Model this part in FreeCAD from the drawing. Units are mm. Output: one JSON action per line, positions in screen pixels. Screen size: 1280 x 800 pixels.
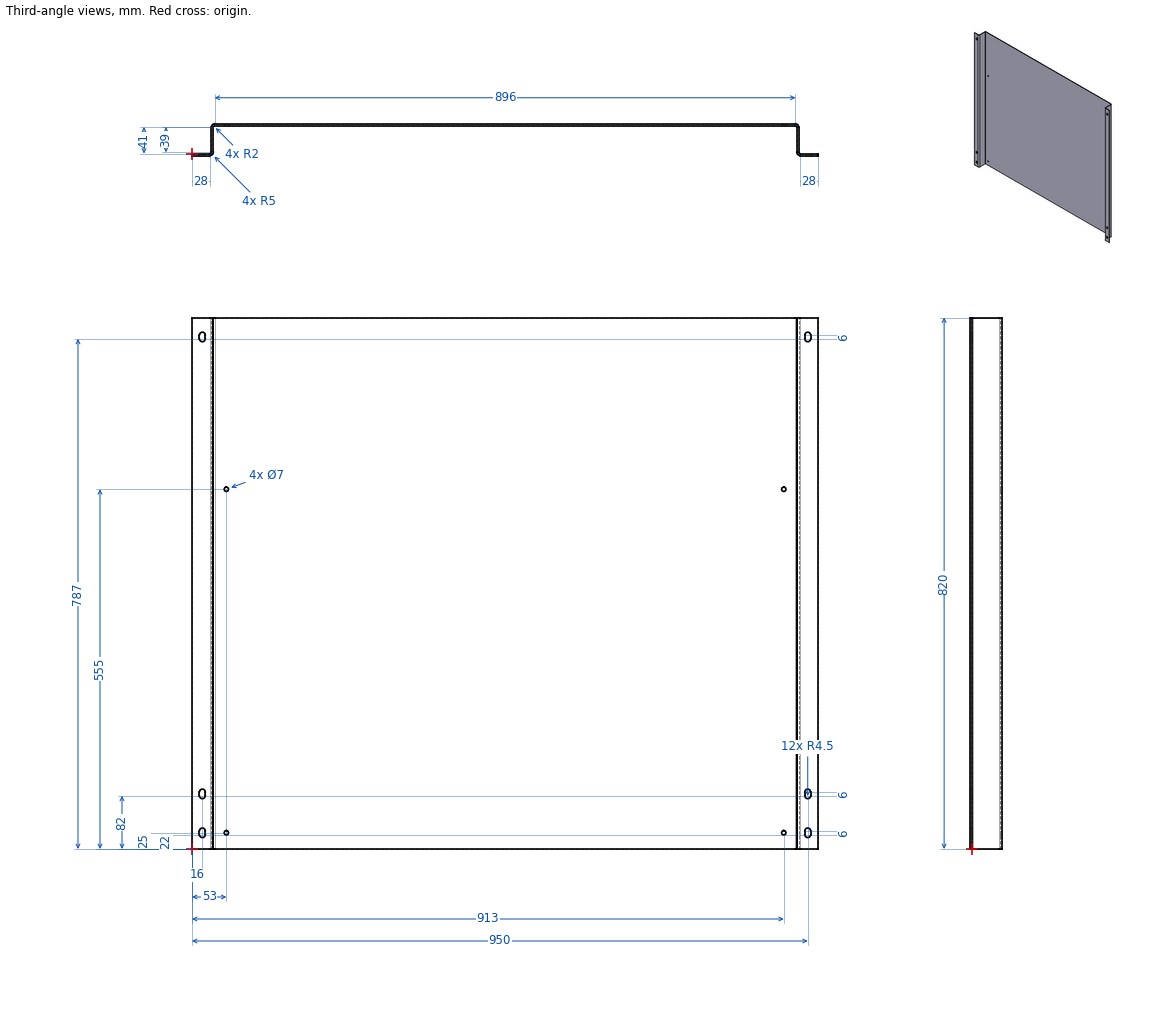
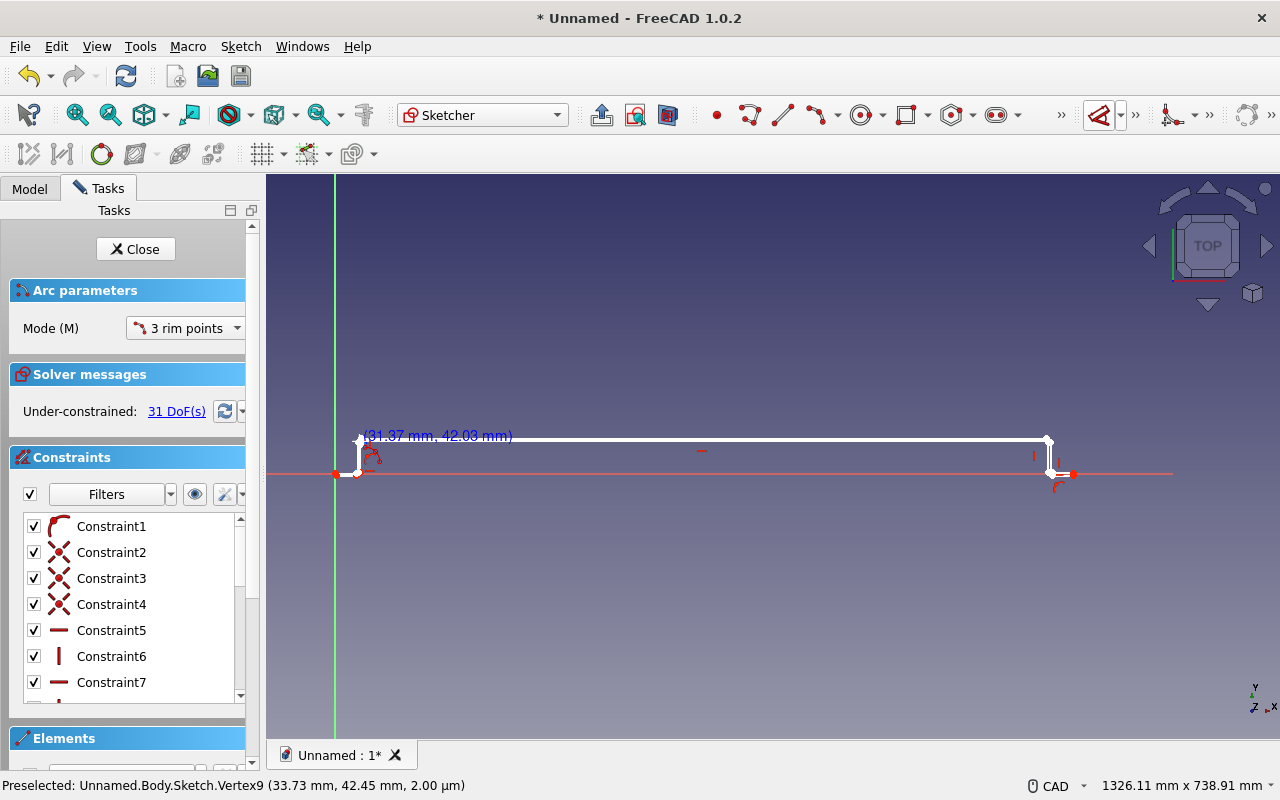
{"action": "scroll", "coordinate": [1047, 441], "scroll_direction": "up", "scroll_amount": 10}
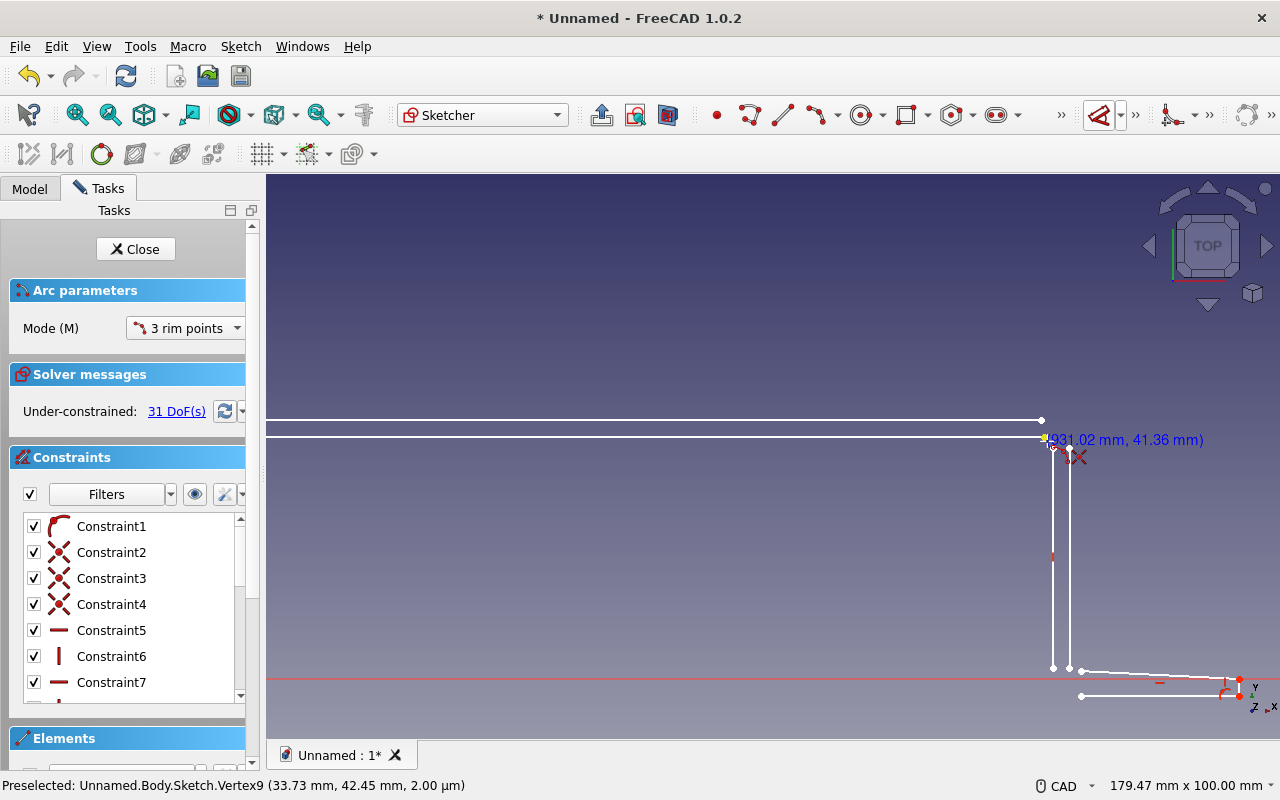
{"action": "left_click", "coordinate": [1044, 437]}
{"action": "left_click", "coordinate": [1053, 448]}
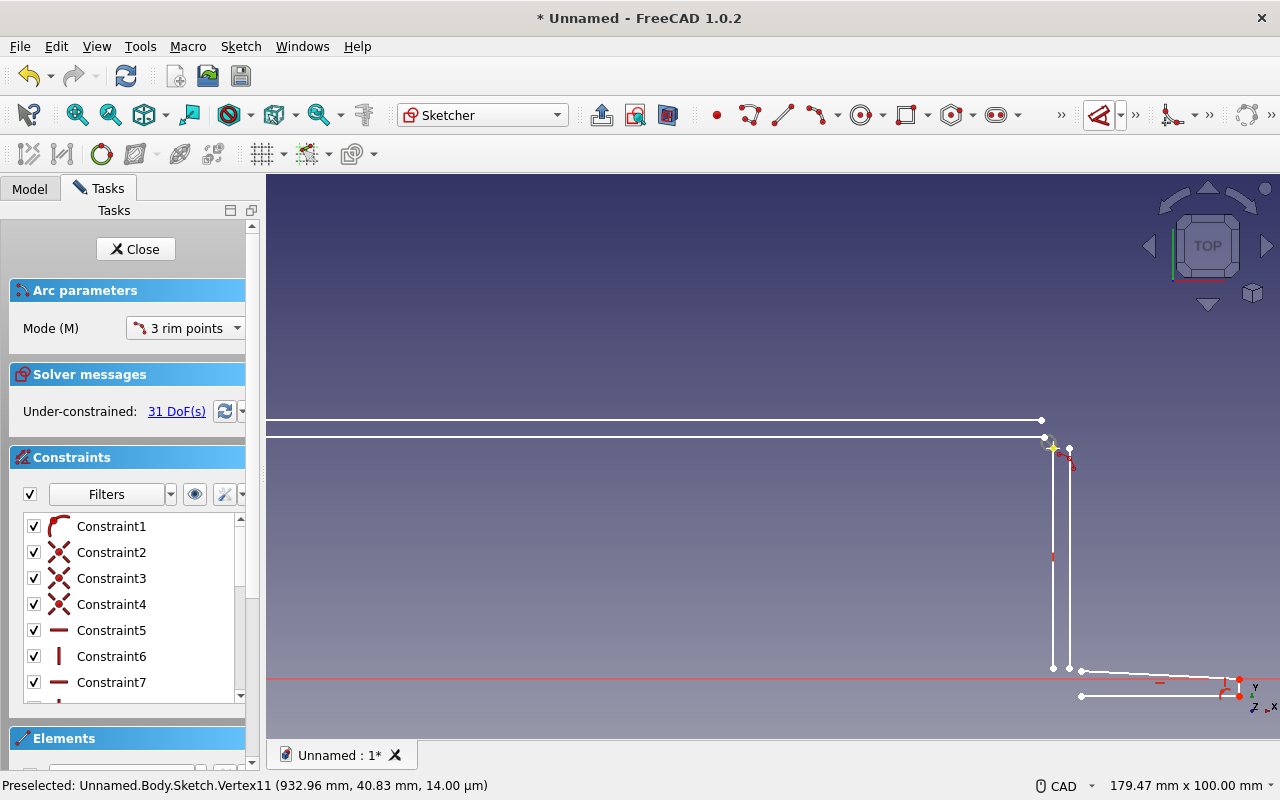
{"action": "scroll", "coordinate": [1050, 439], "scroll_direction": "up", "scroll_amount": 8}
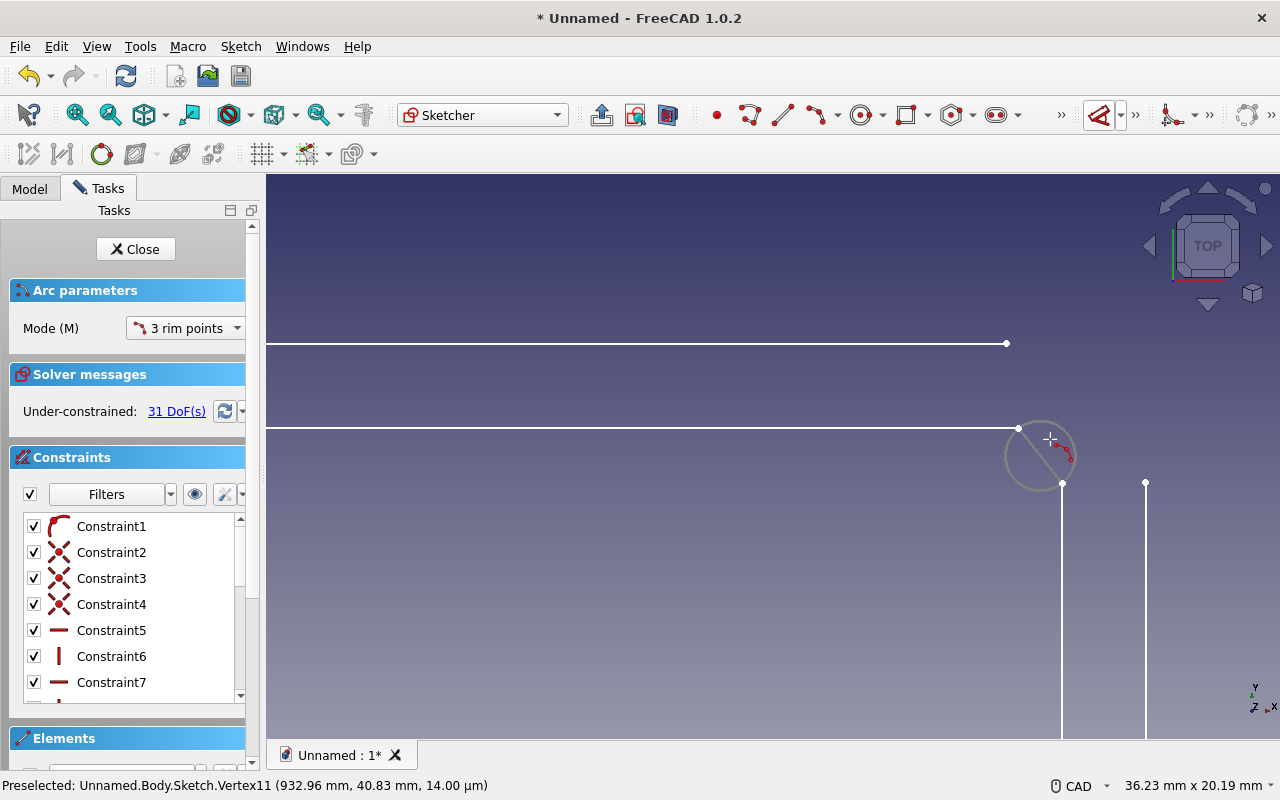
{"action": "left_click", "coordinate": [1047, 439]}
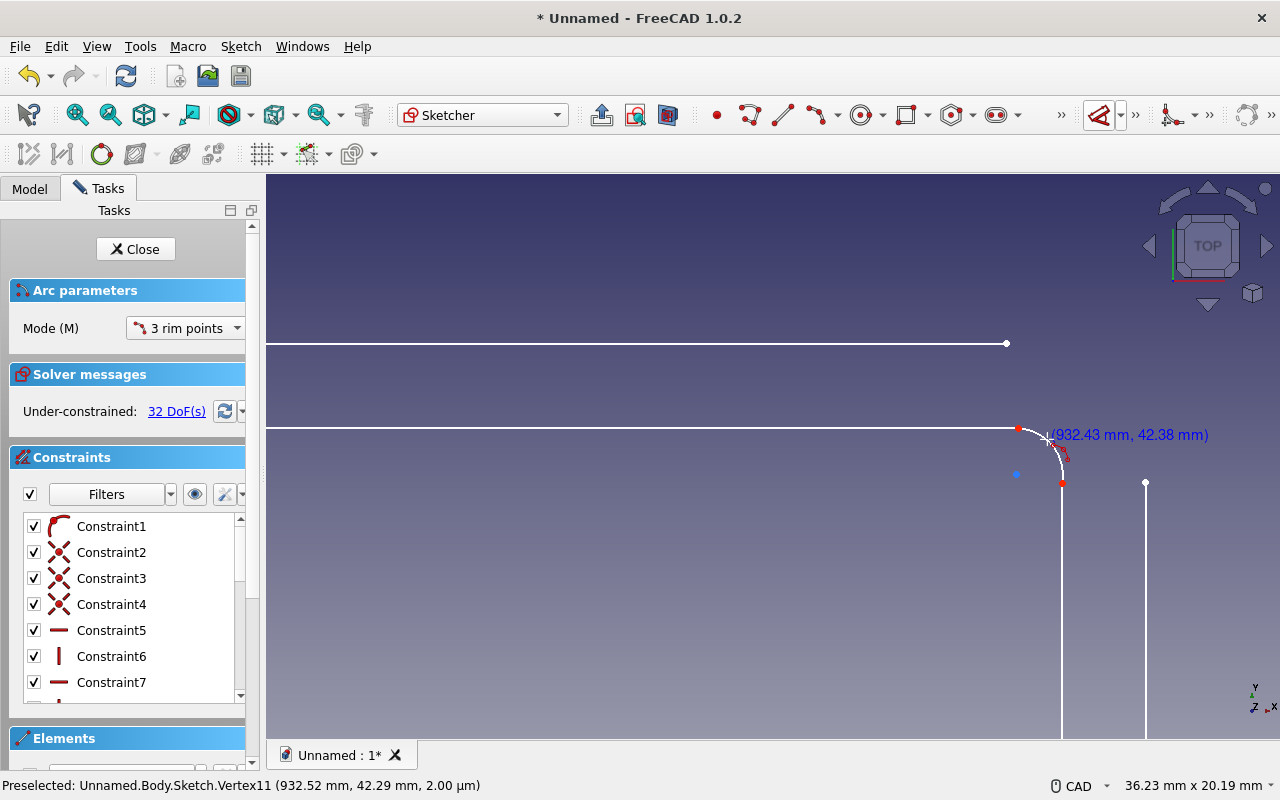
{"action": "scroll", "coordinate": [1048, 441], "scroll_direction": "down", "scroll_amount": 18}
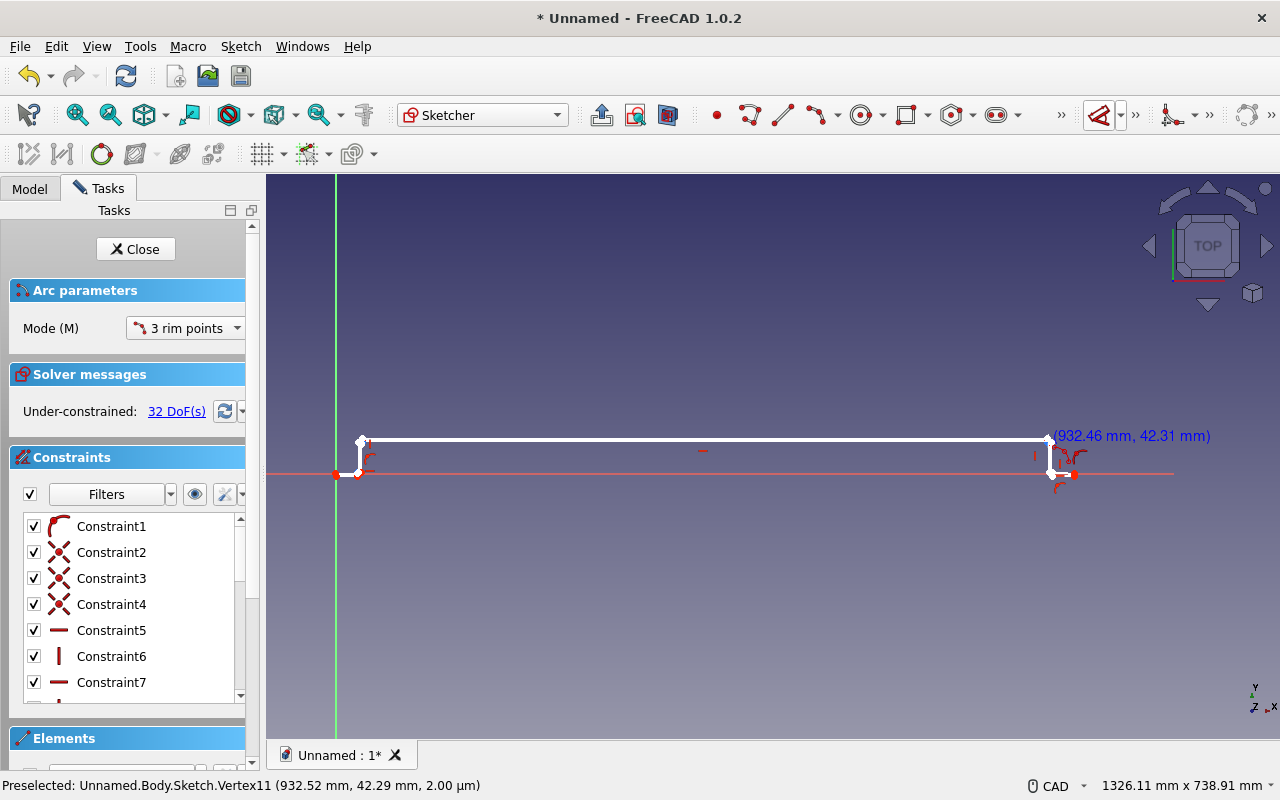
{"action": "scroll", "coordinate": [1049, 472], "scroll_direction": "up", "scroll_amount": 12}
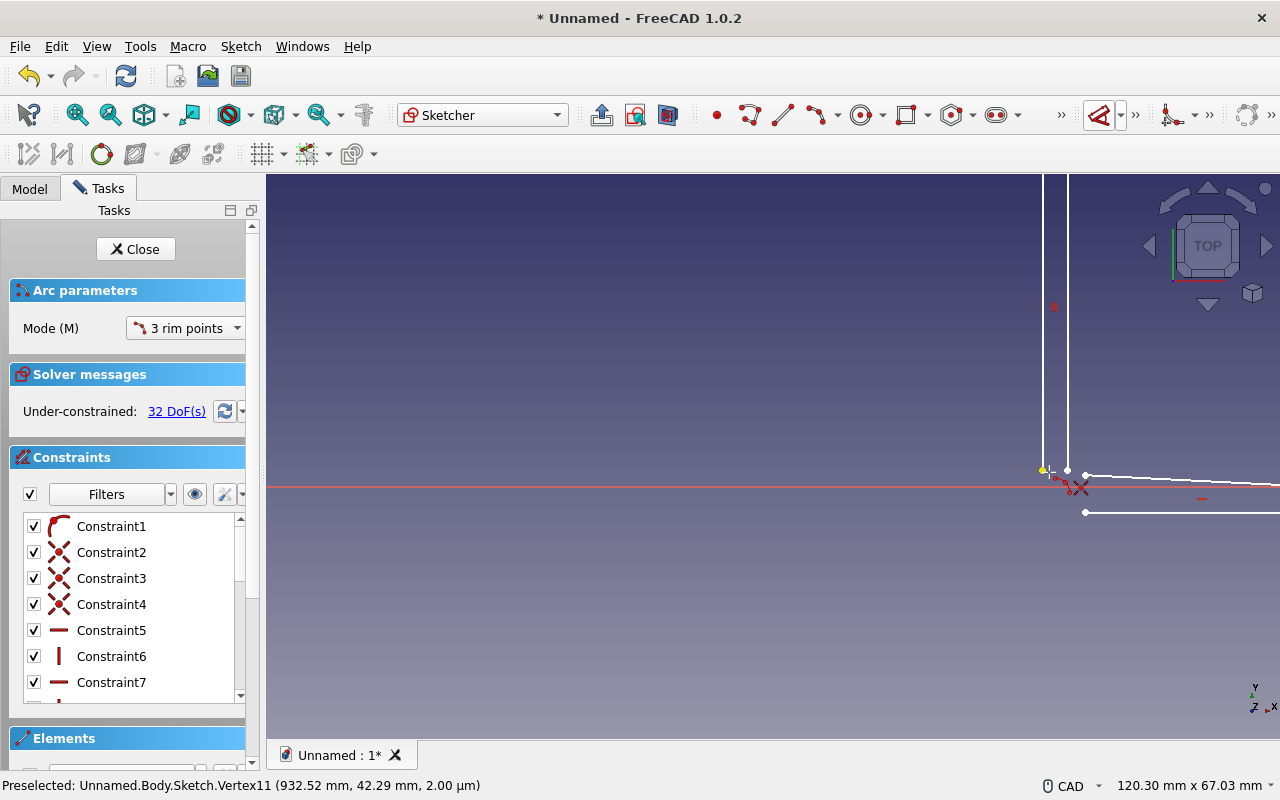
{"action": "left_click", "coordinate": [1043, 471]}
{"action": "left_click", "coordinate": [1085, 513]}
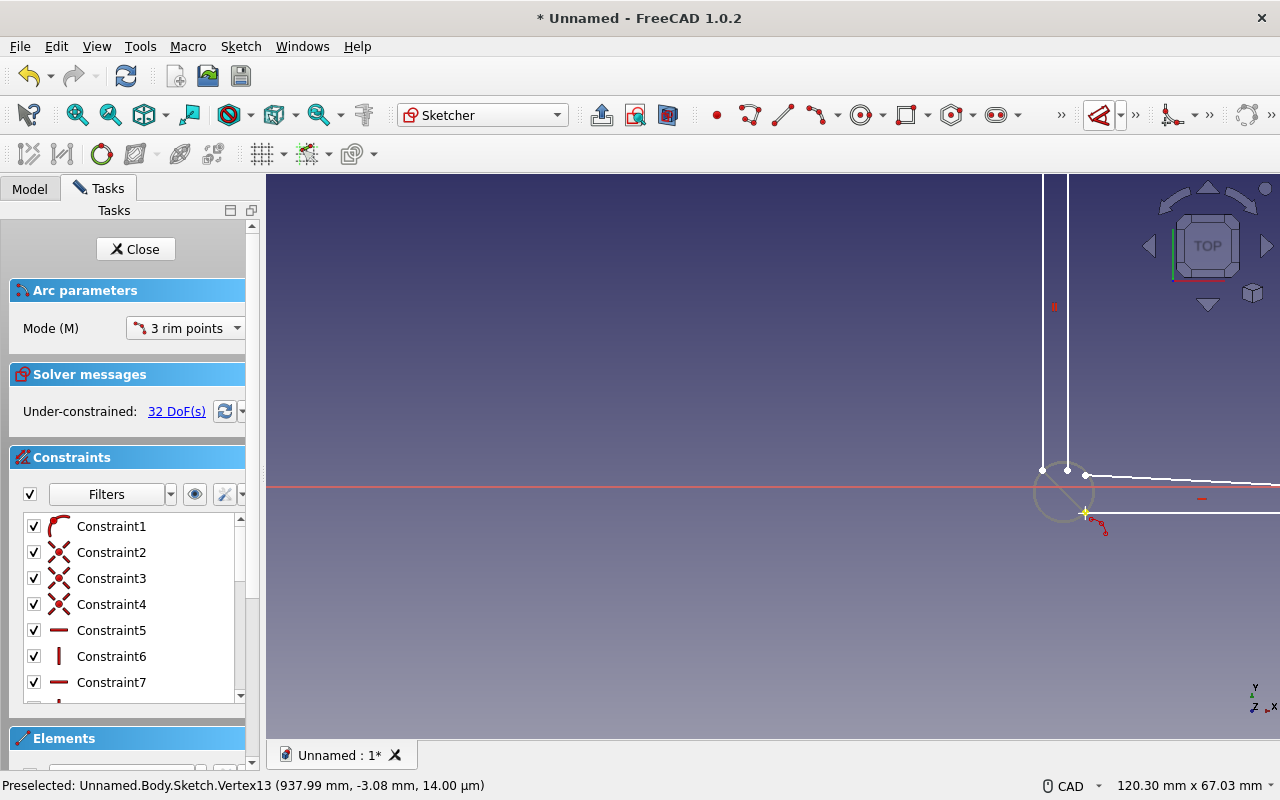
{"action": "scroll", "coordinate": [1055, 500], "scroll_direction": "up", "scroll_amount": 2}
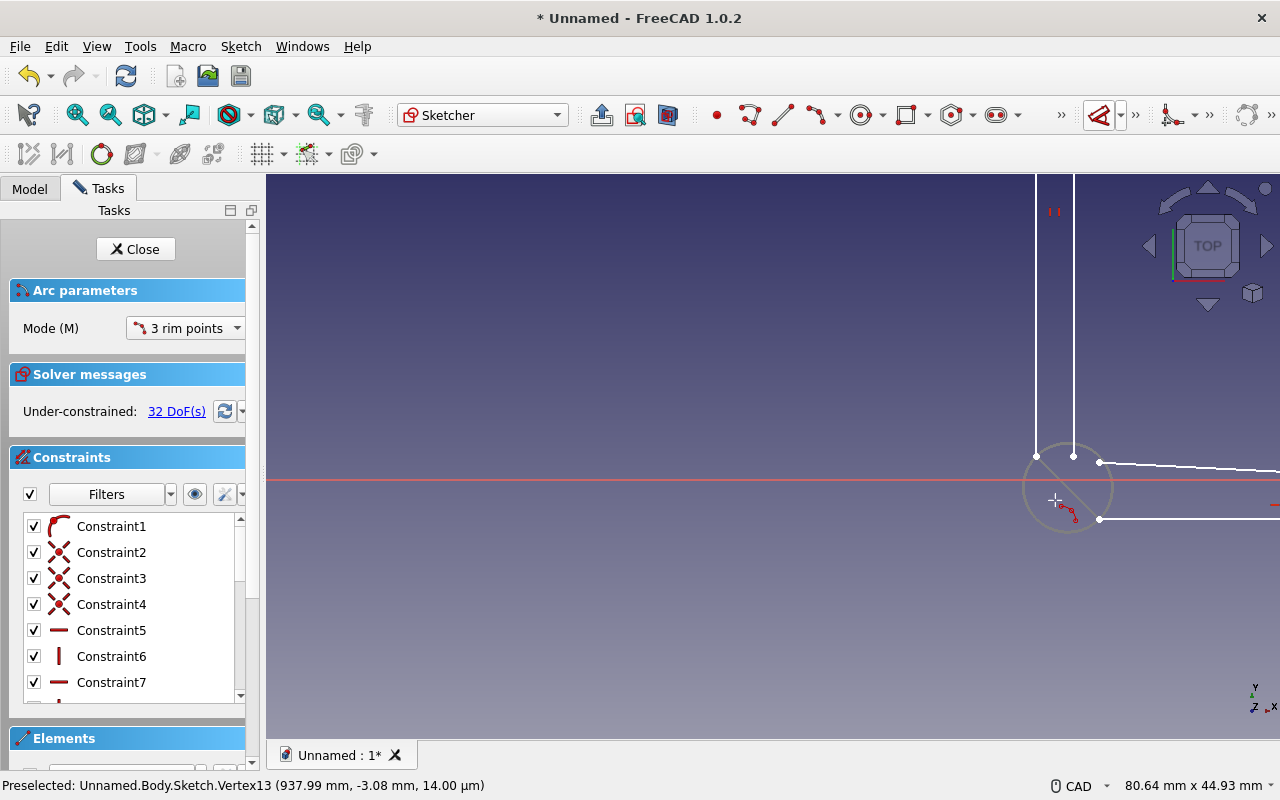
{"action": "left_click", "coordinate": [1055, 500]}